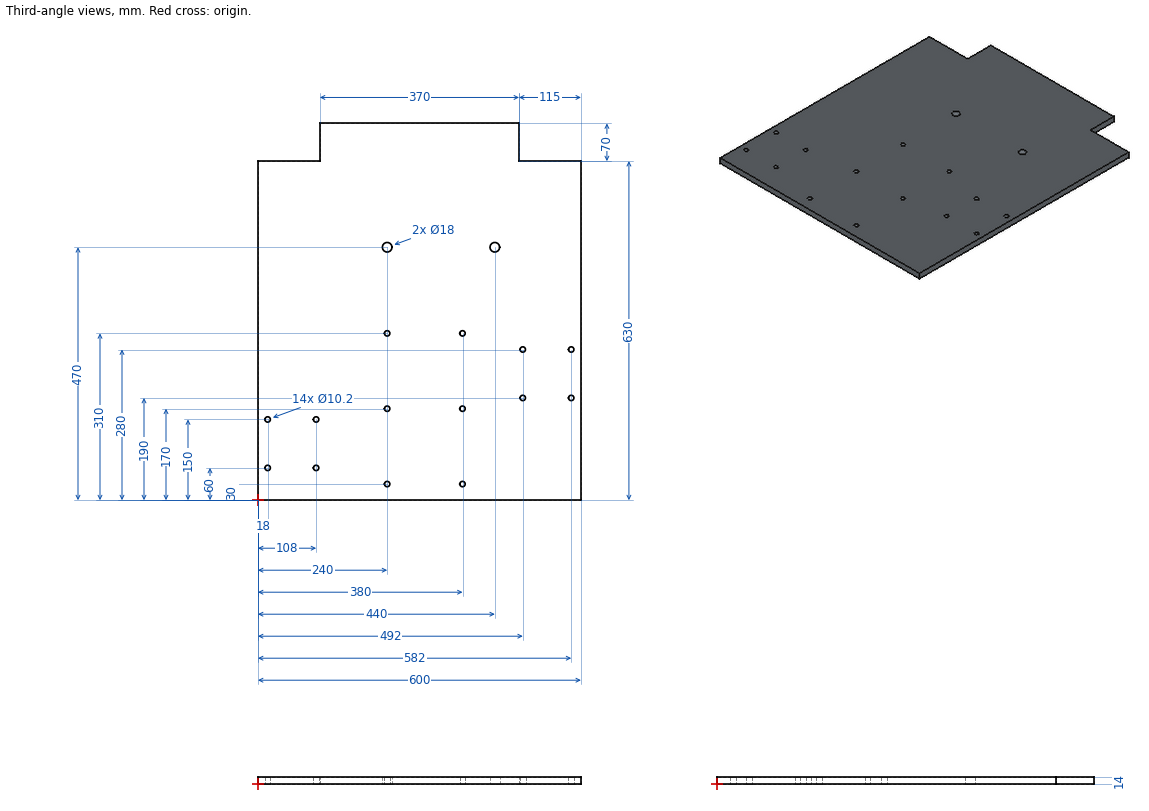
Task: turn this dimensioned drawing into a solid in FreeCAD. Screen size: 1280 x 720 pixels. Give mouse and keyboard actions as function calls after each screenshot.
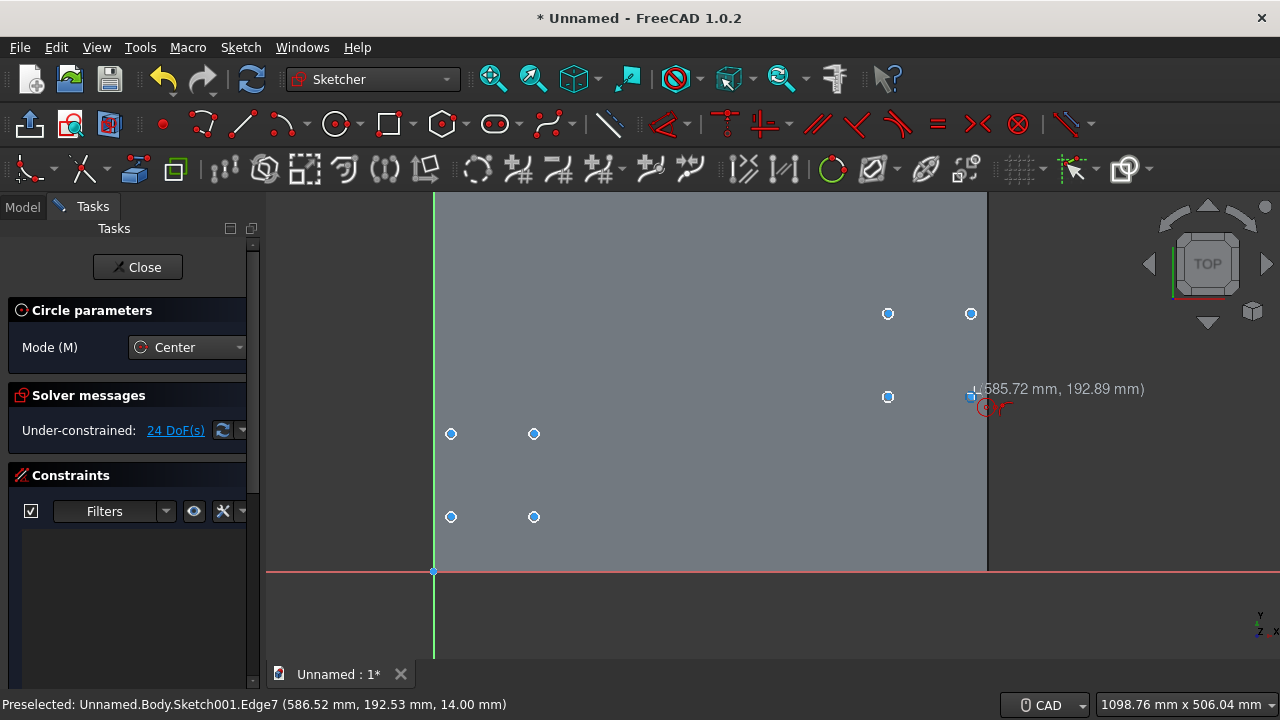
scroll(655, 285, up, 8)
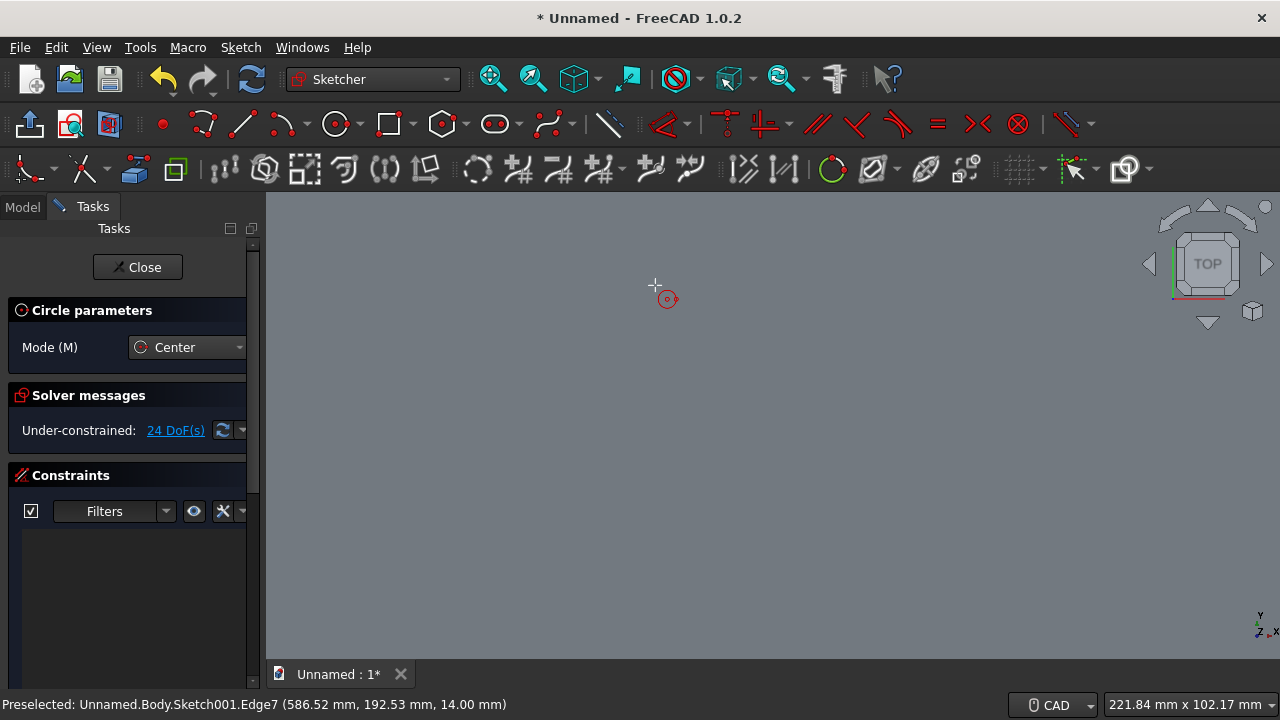
scroll(655, 284, down, 8)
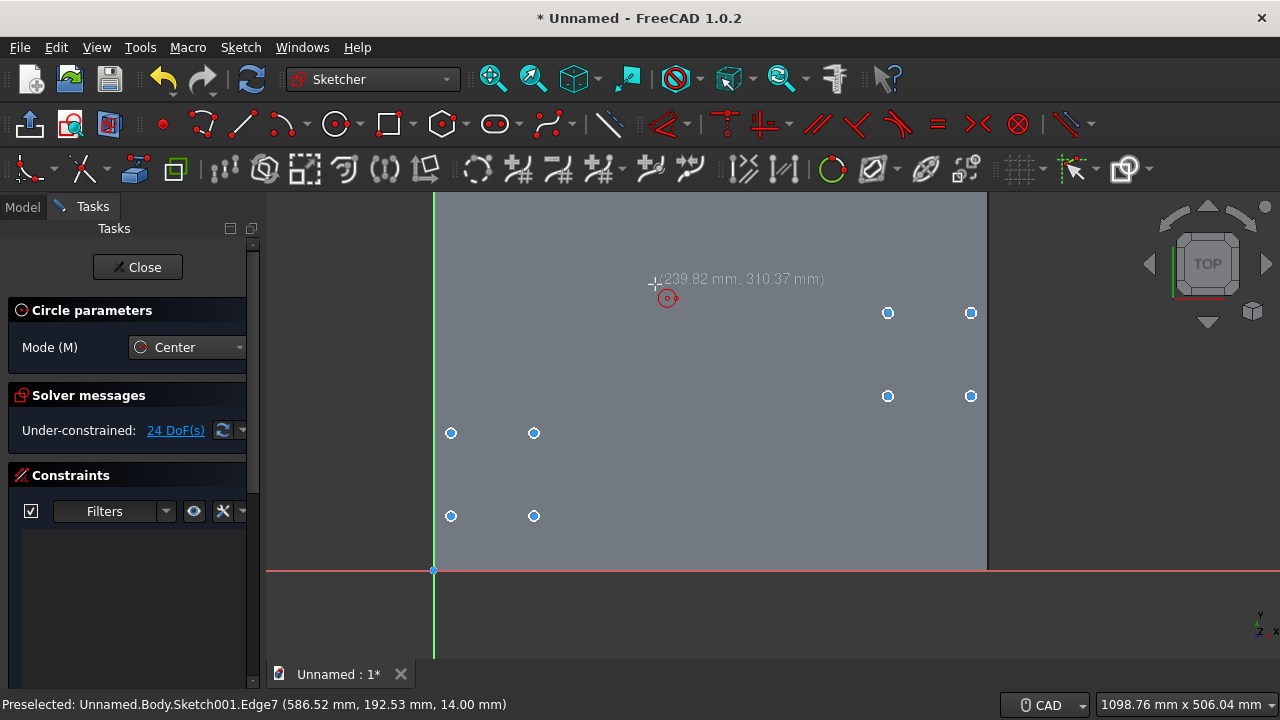
click(655, 285)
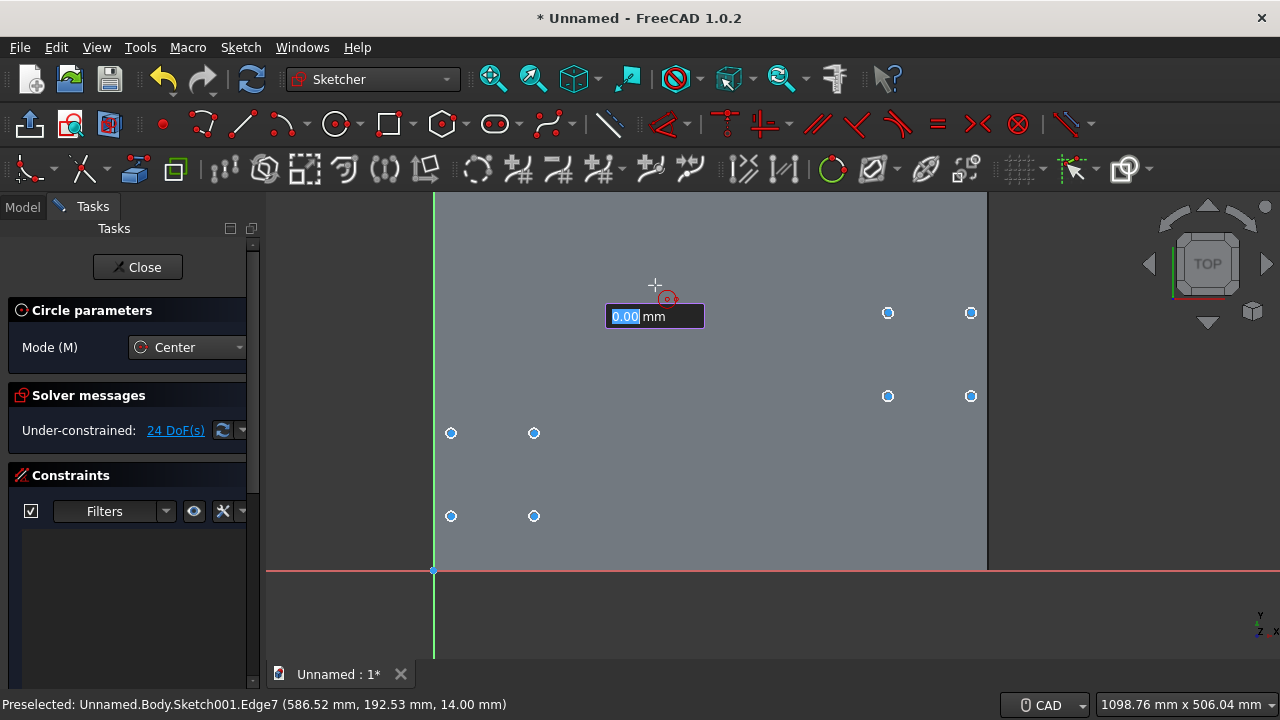
scroll(659, 281, up, 7)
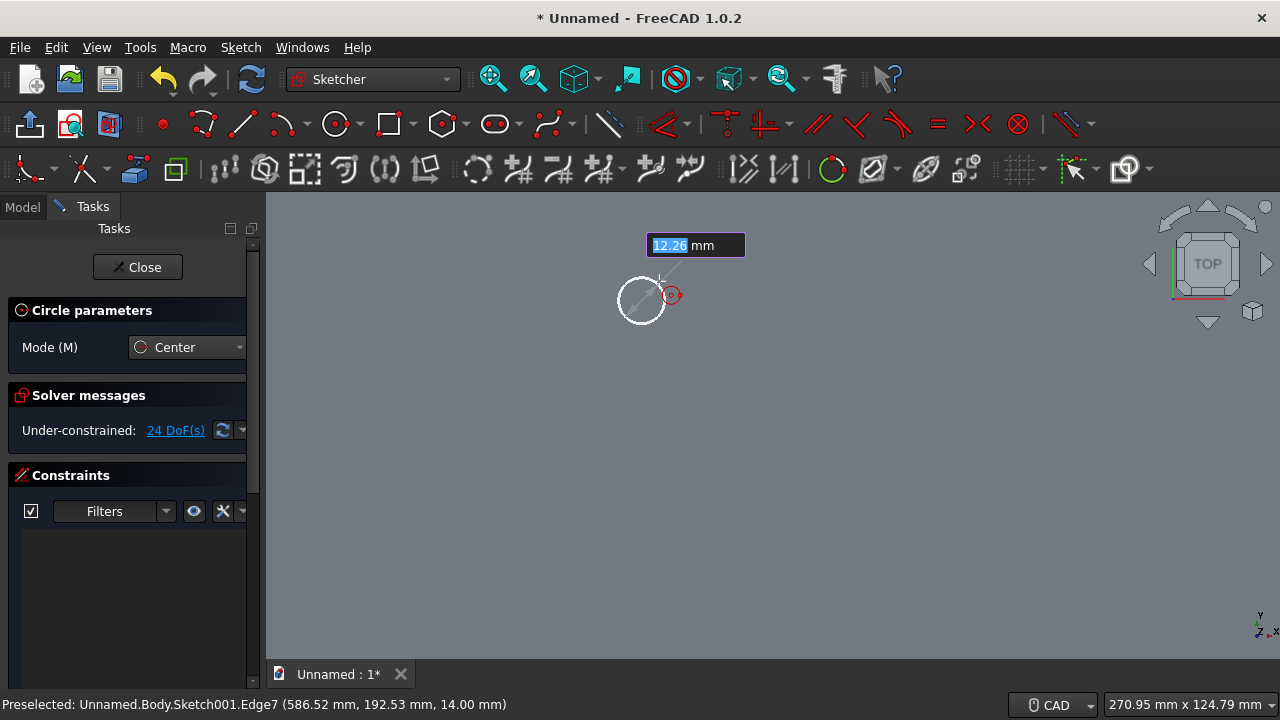
click(657, 282)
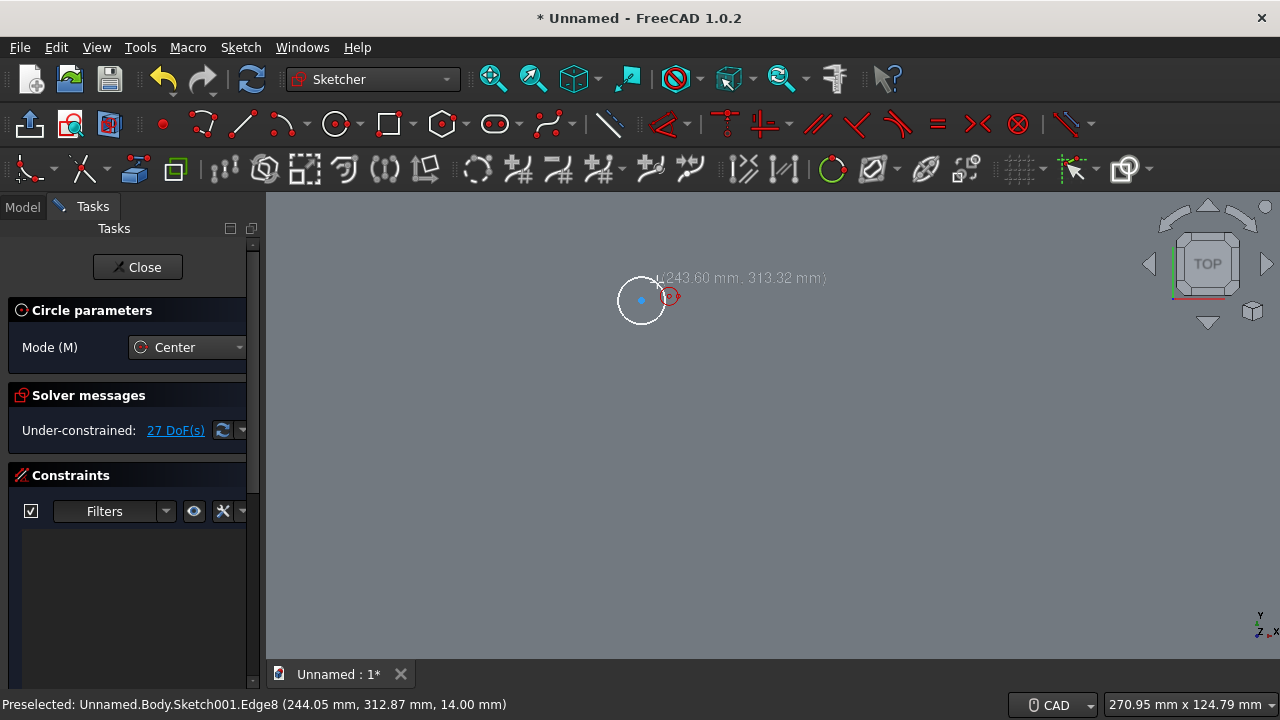
scroll(659, 281, down, 7)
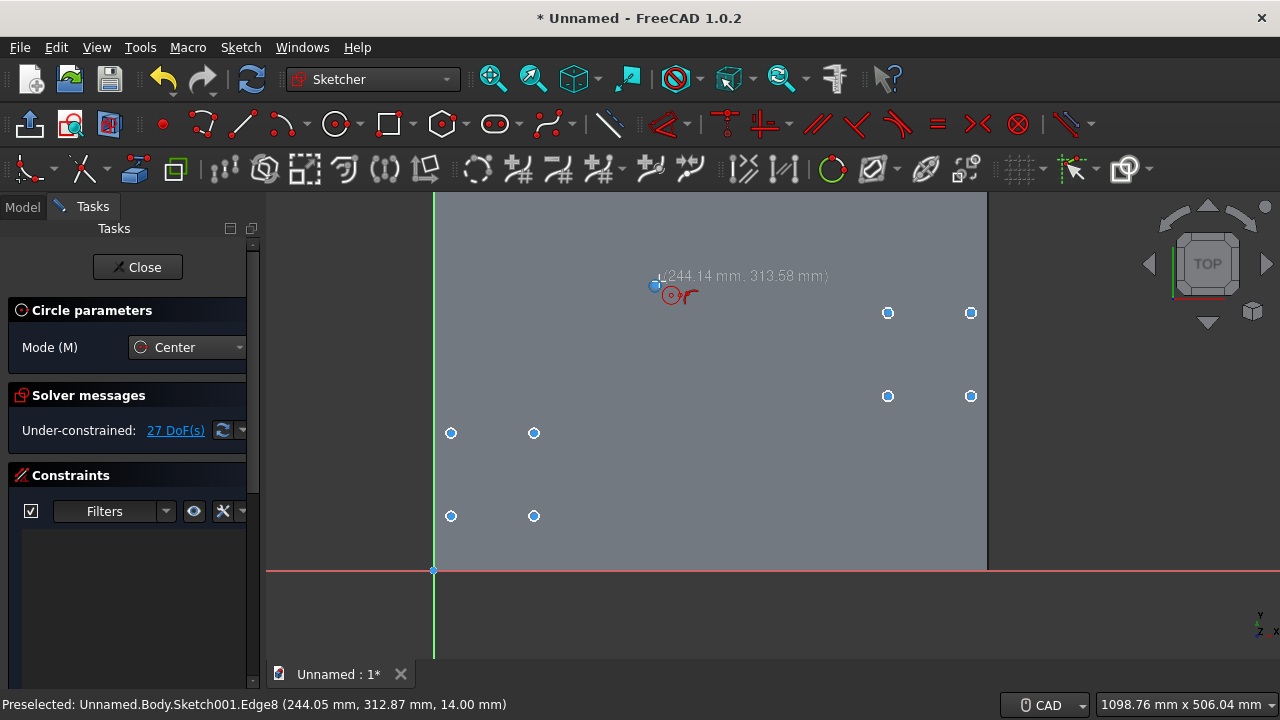
scroll(785, 285, up, 8)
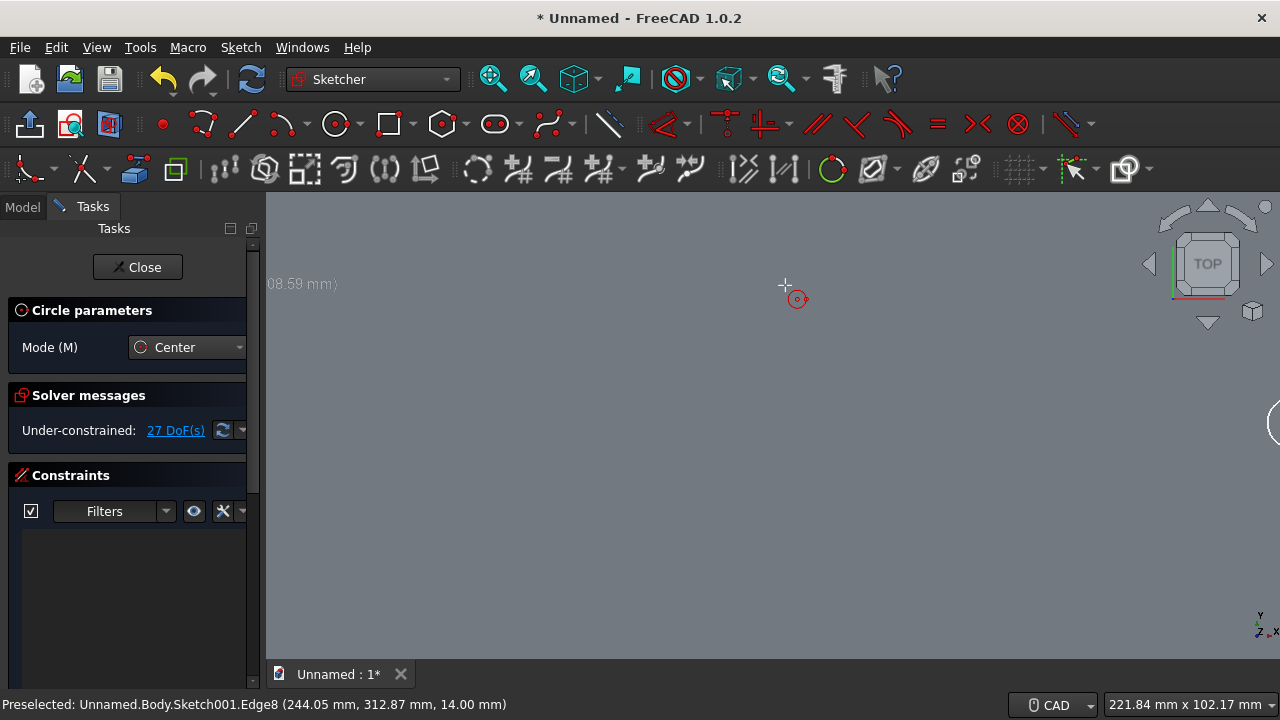
scroll(785, 285, down, 8)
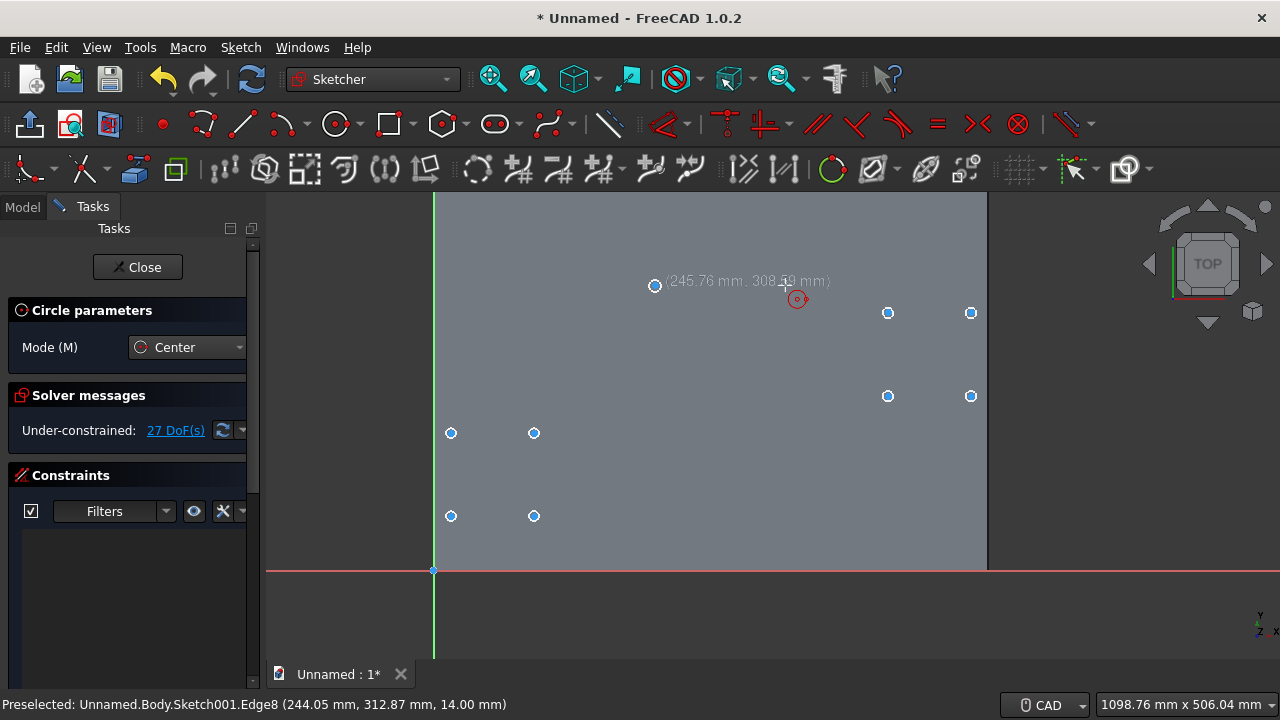
click(785, 285)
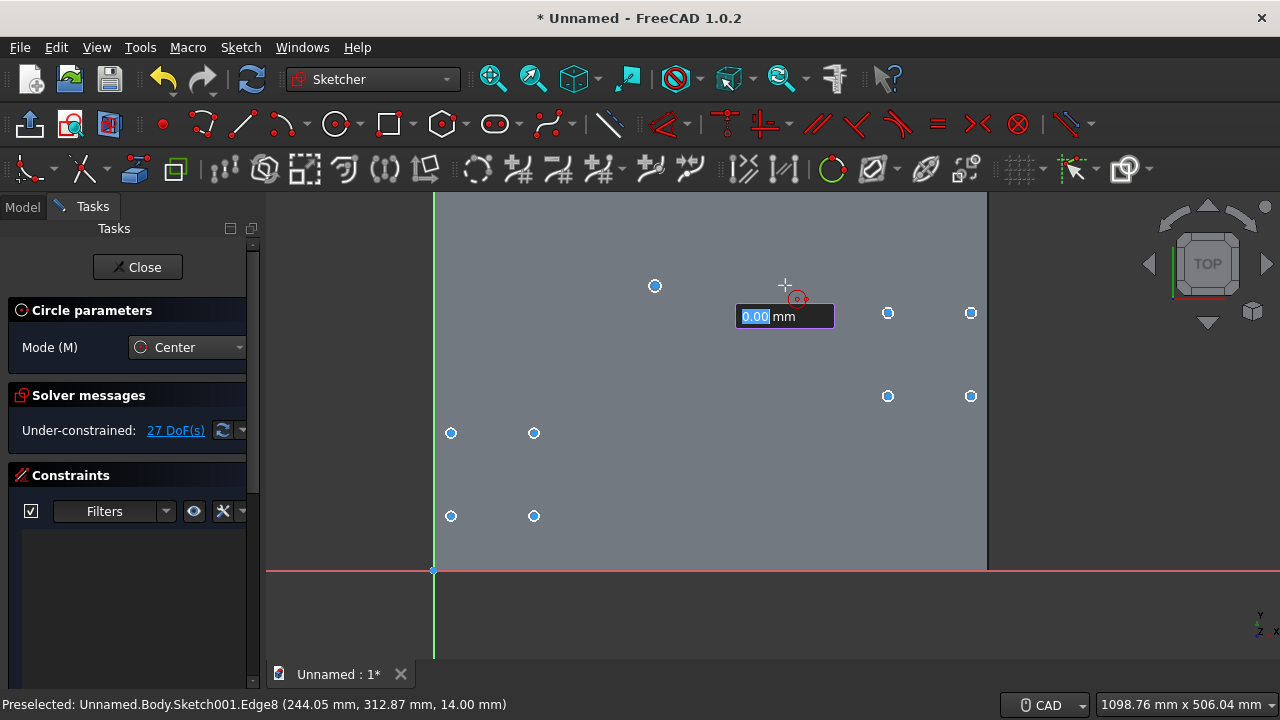
scroll(788, 281, up, 7)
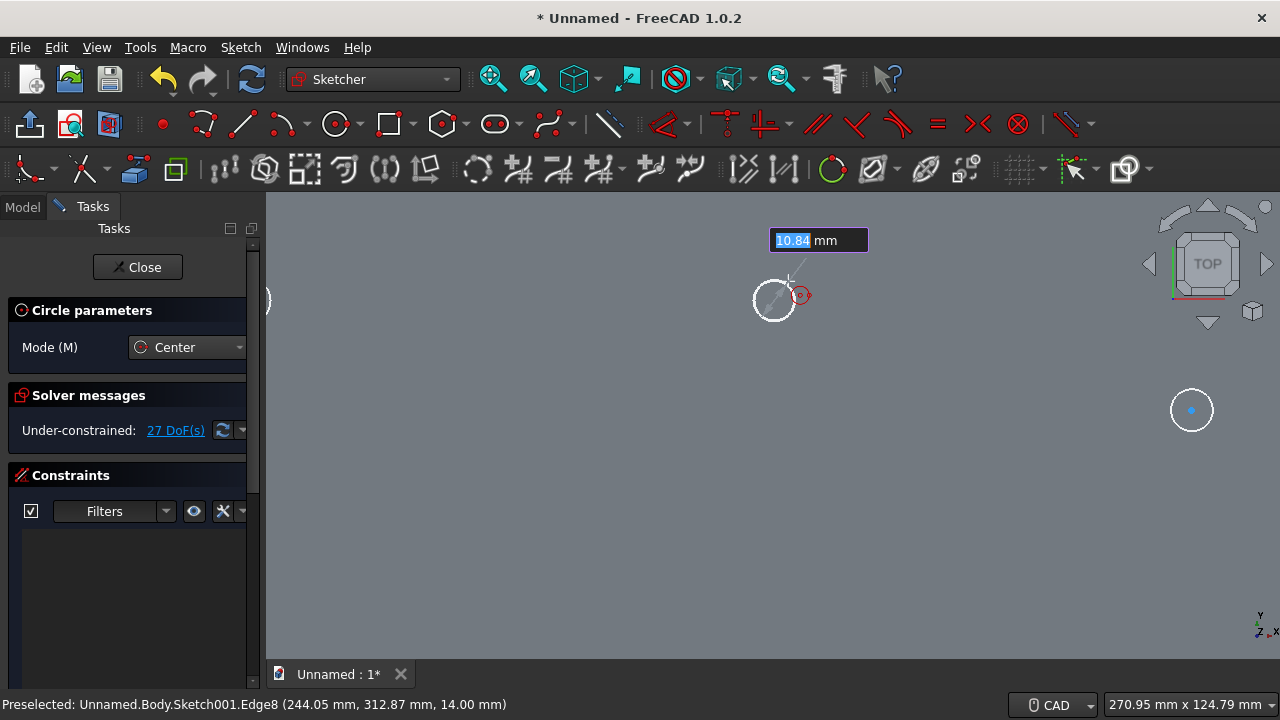
click(786, 282)